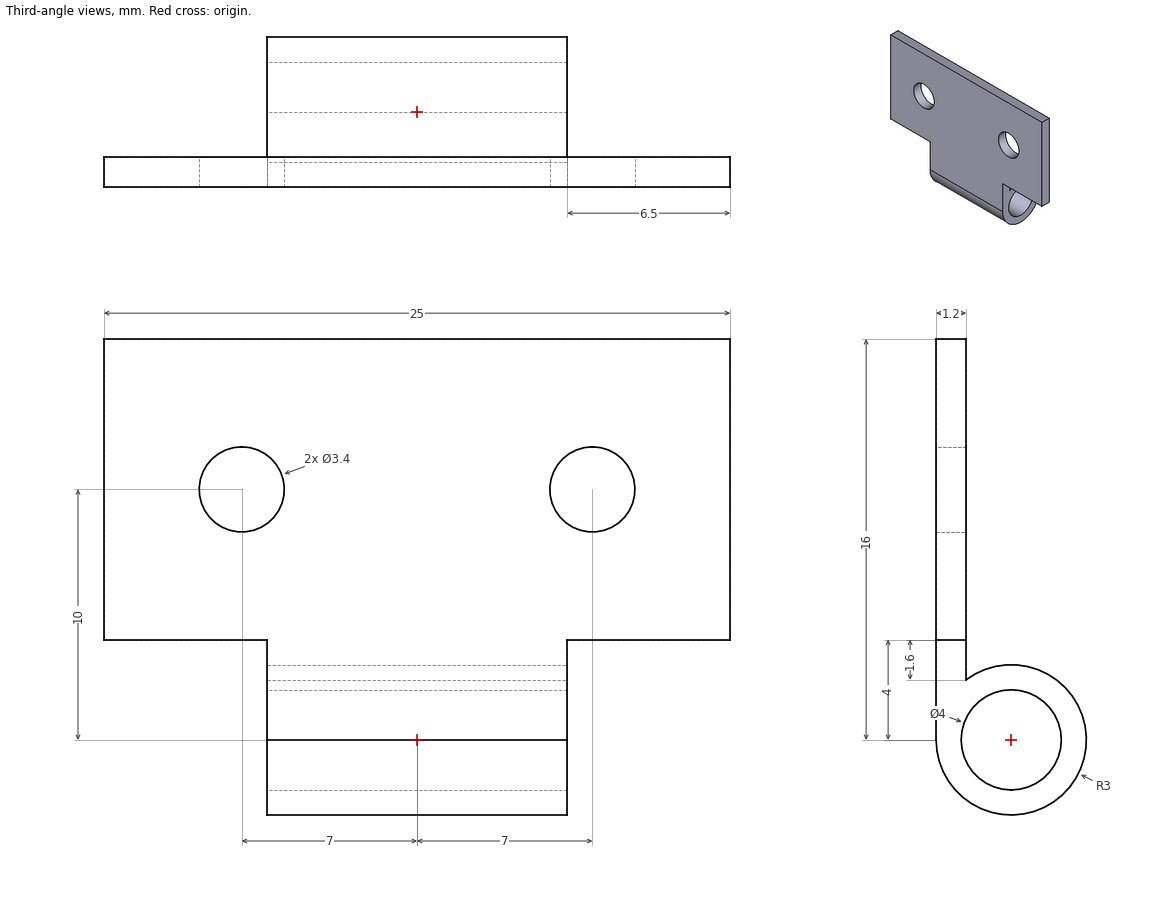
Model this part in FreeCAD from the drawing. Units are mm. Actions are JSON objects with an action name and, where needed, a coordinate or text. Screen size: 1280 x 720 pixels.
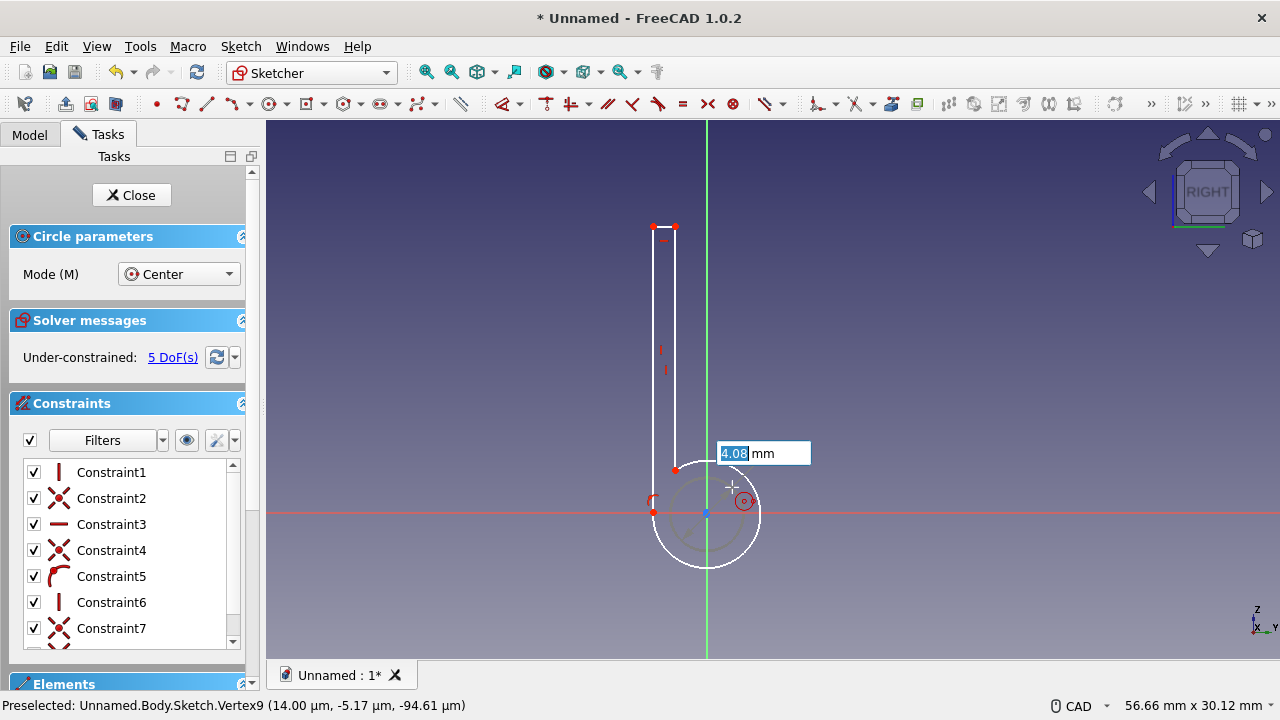
{"action": "type", "text": "4"}
{"action": "key", "text": "Return"}
{"action": "key", "text": "Escape"}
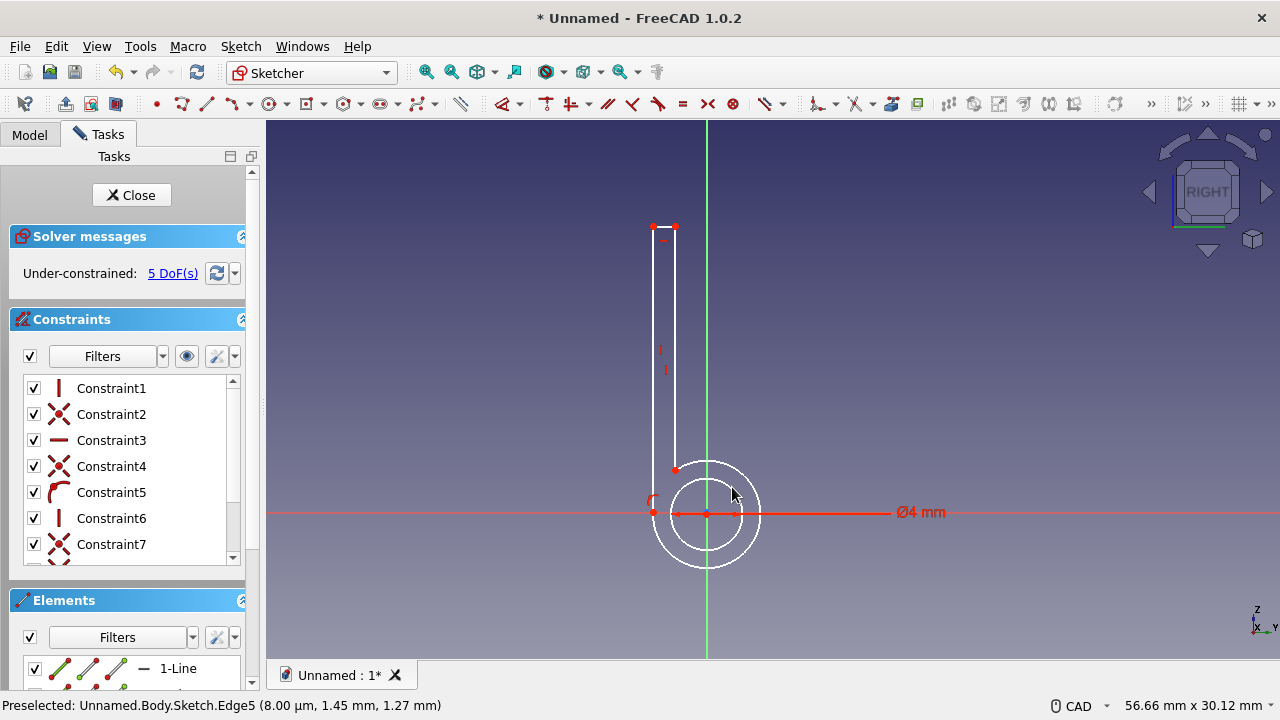
{"action": "left_click", "coordinate": [653, 313]}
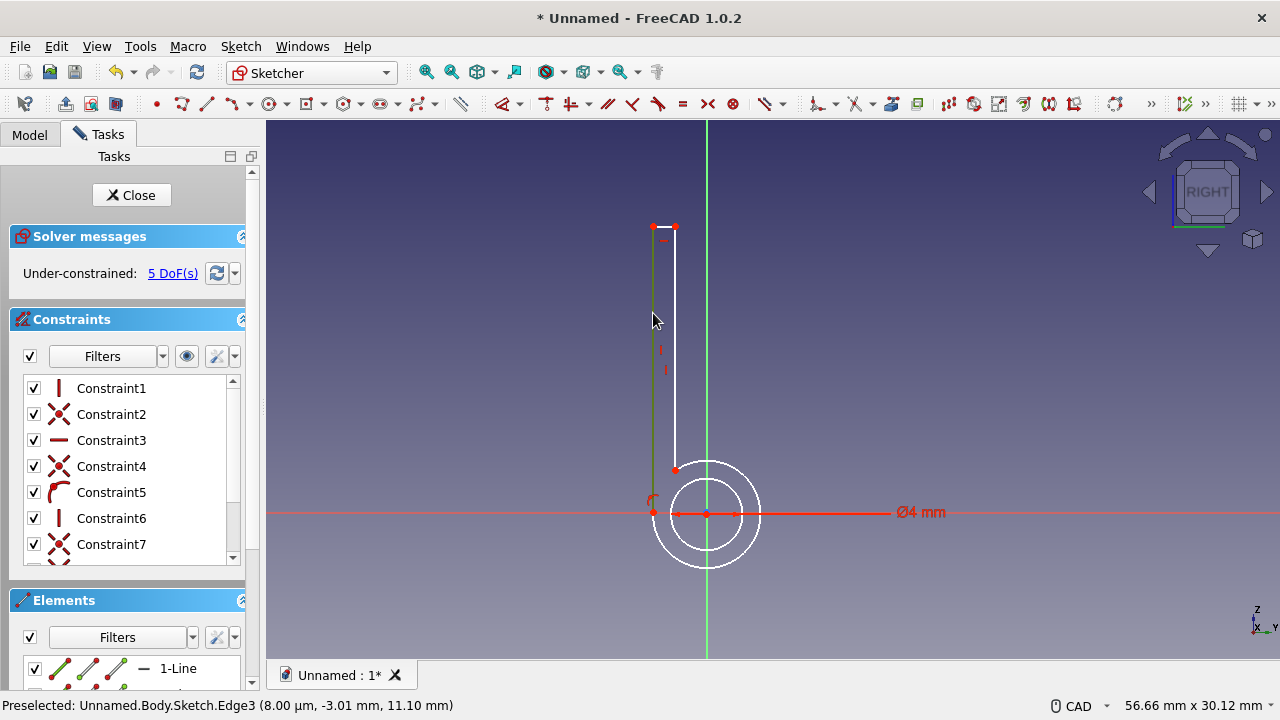
{"action": "left_click", "coordinate": [707, 568]}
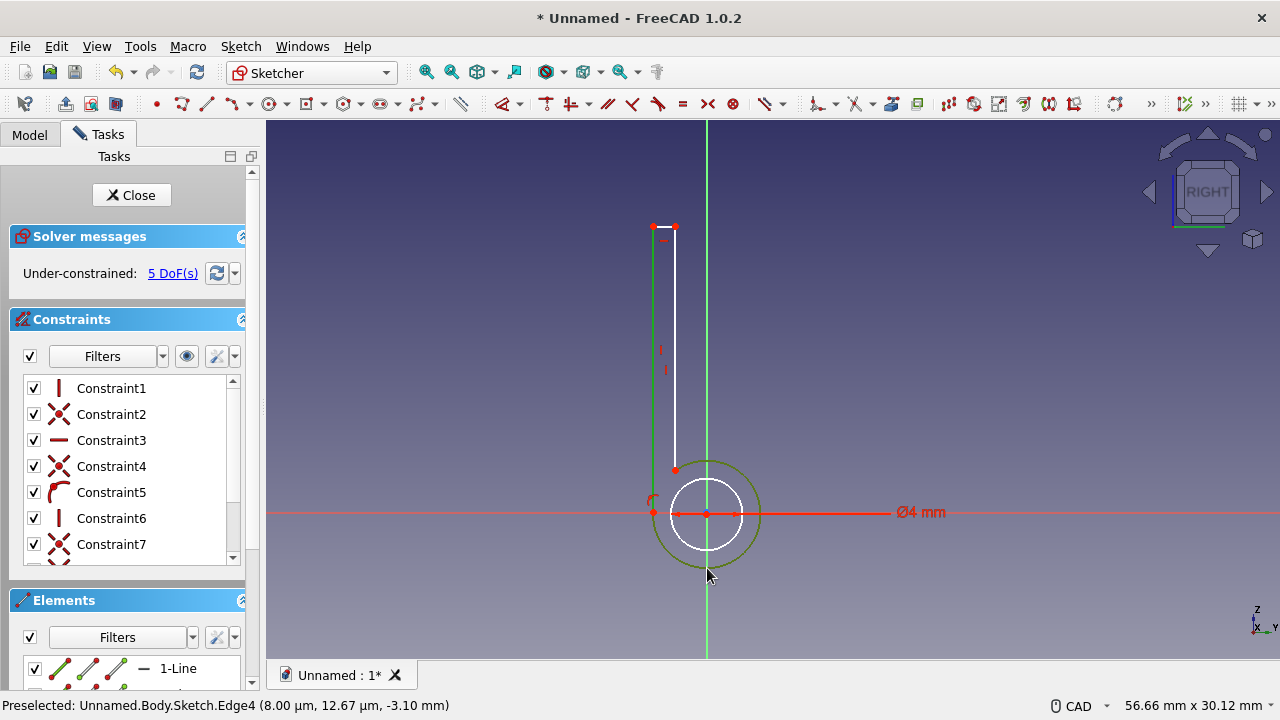
{"action": "left_click", "coordinate": [658, 104]}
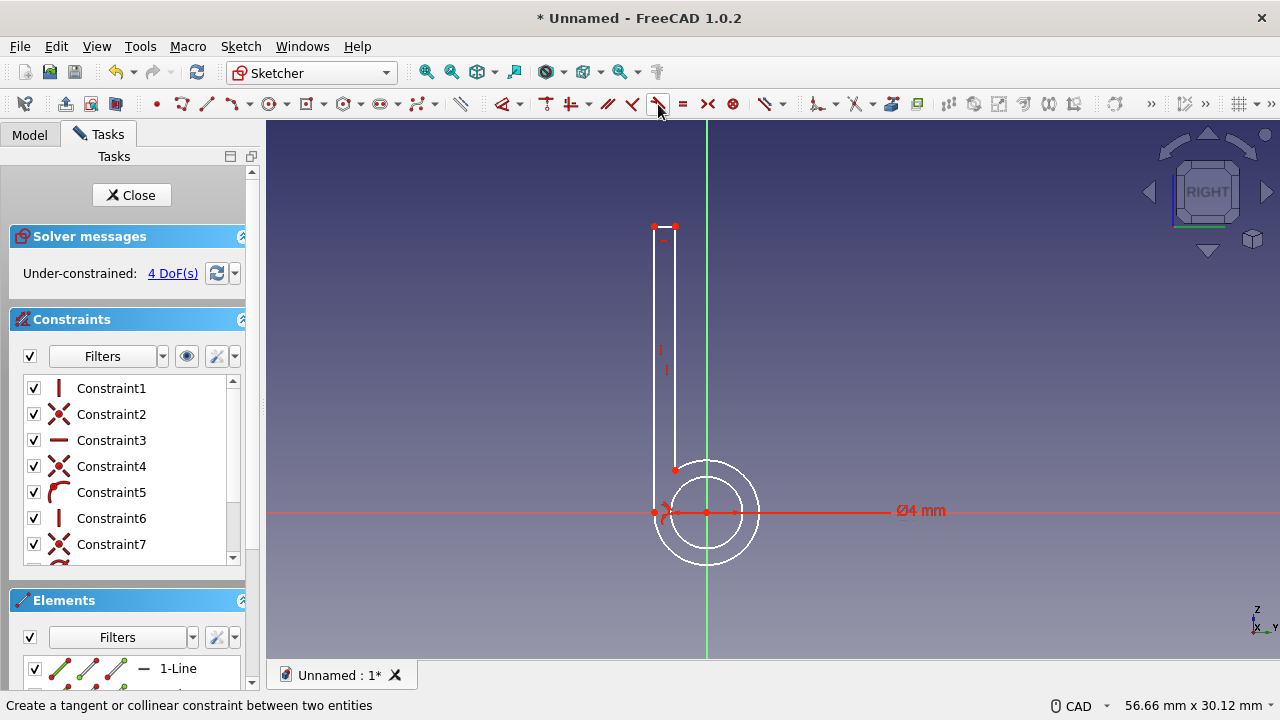
{"action": "left_click", "coordinate": [707, 513]}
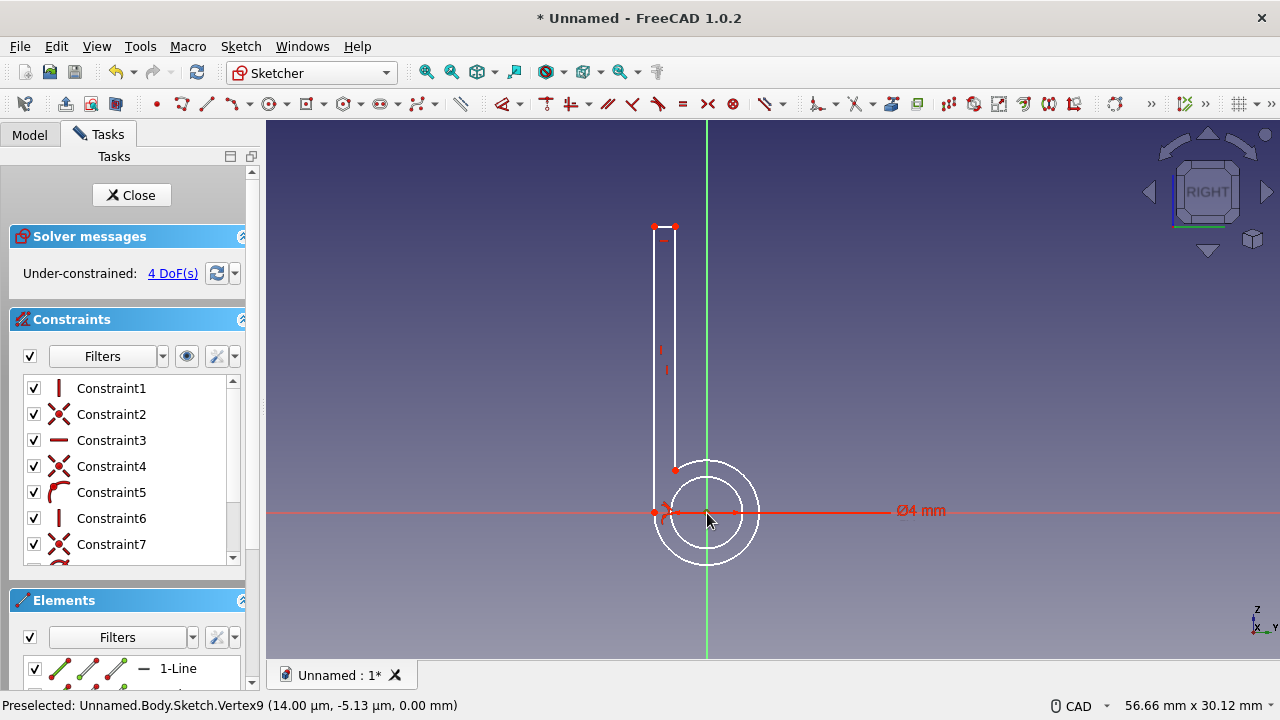
{"action": "left_click", "coordinate": [707, 596]}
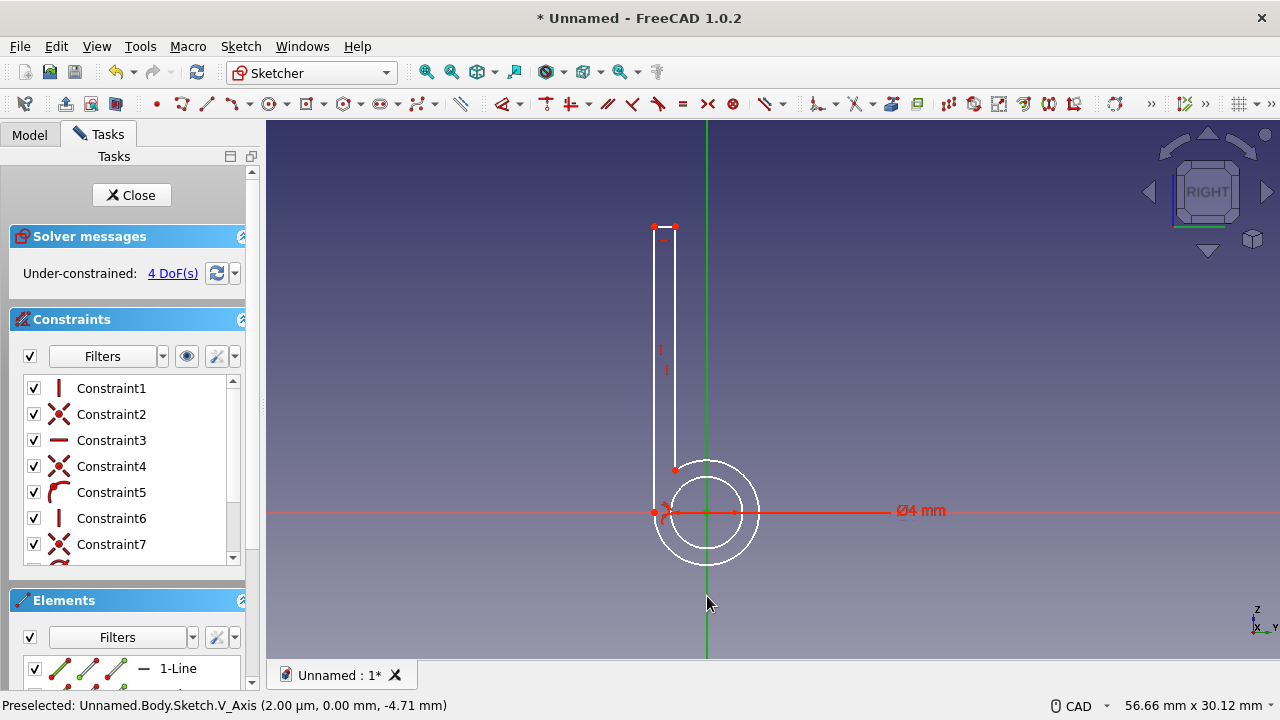
{"action": "left_click", "coordinate": [546, 104]}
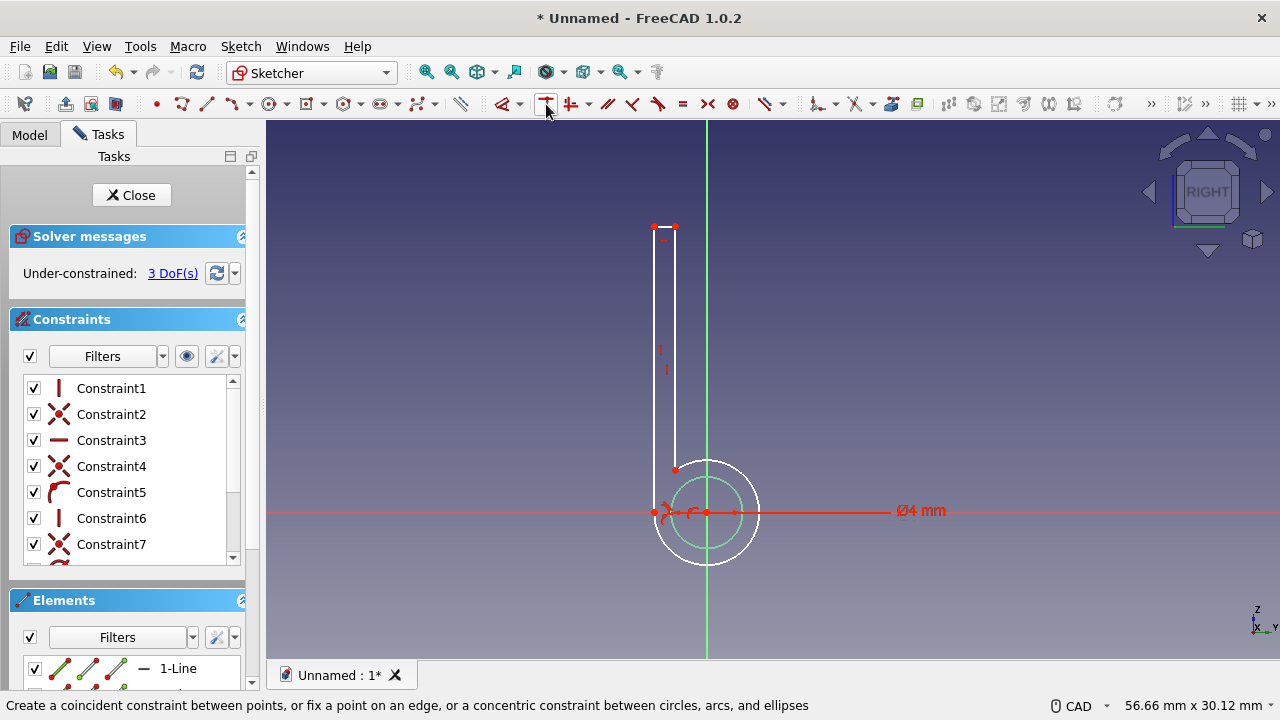
{"action": "left_click", "coordinate": [709, 565]}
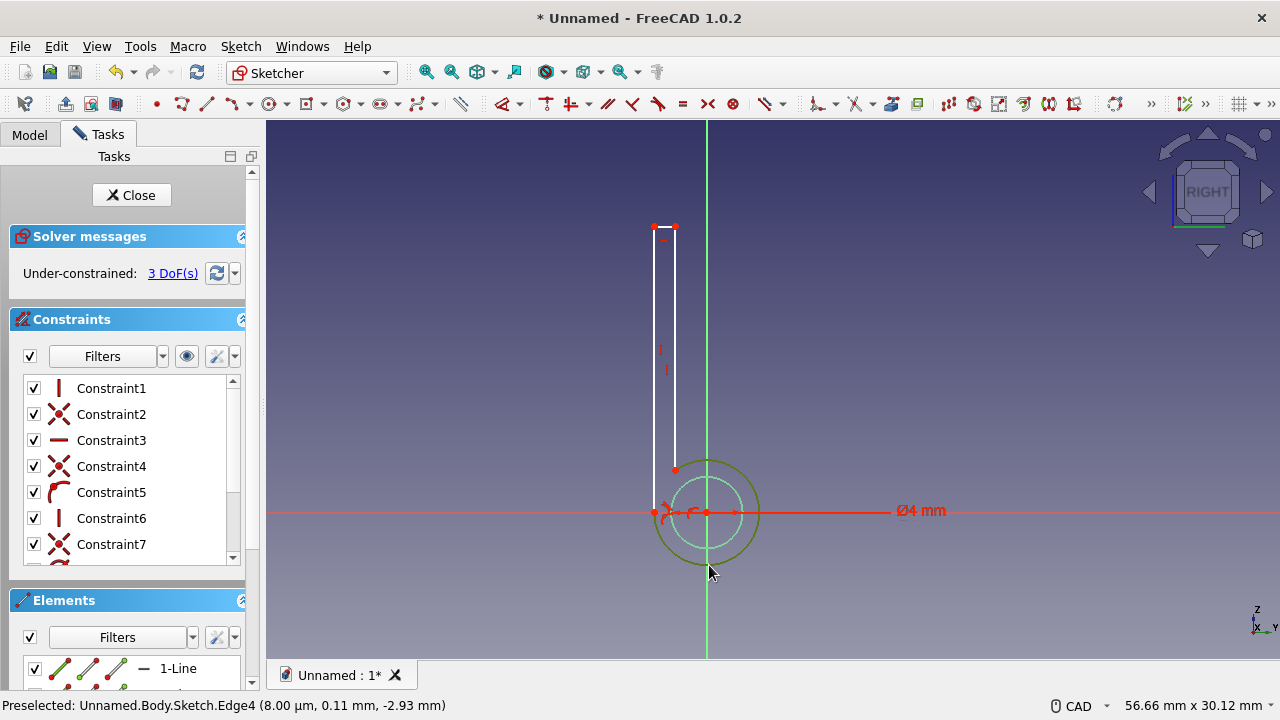
{"action": "left_click", "coordinate": [520, 104]}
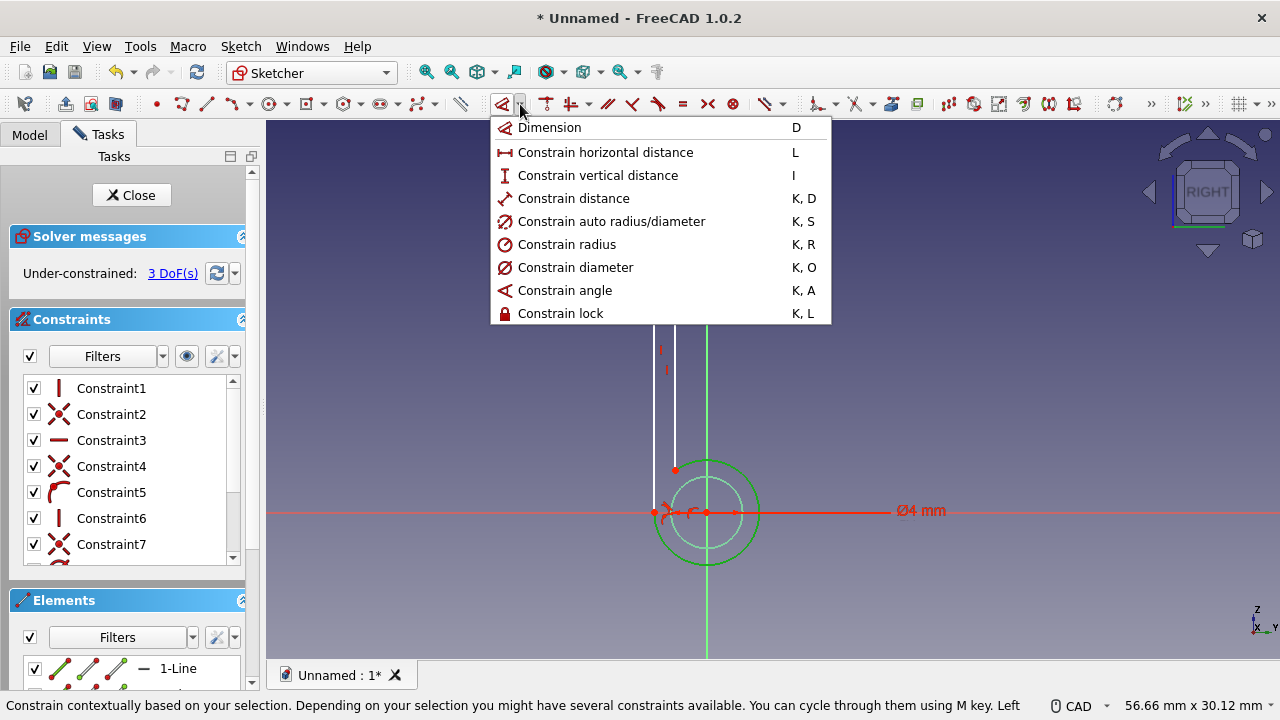
{"action": "left_click", "coordinate": [661, 244]}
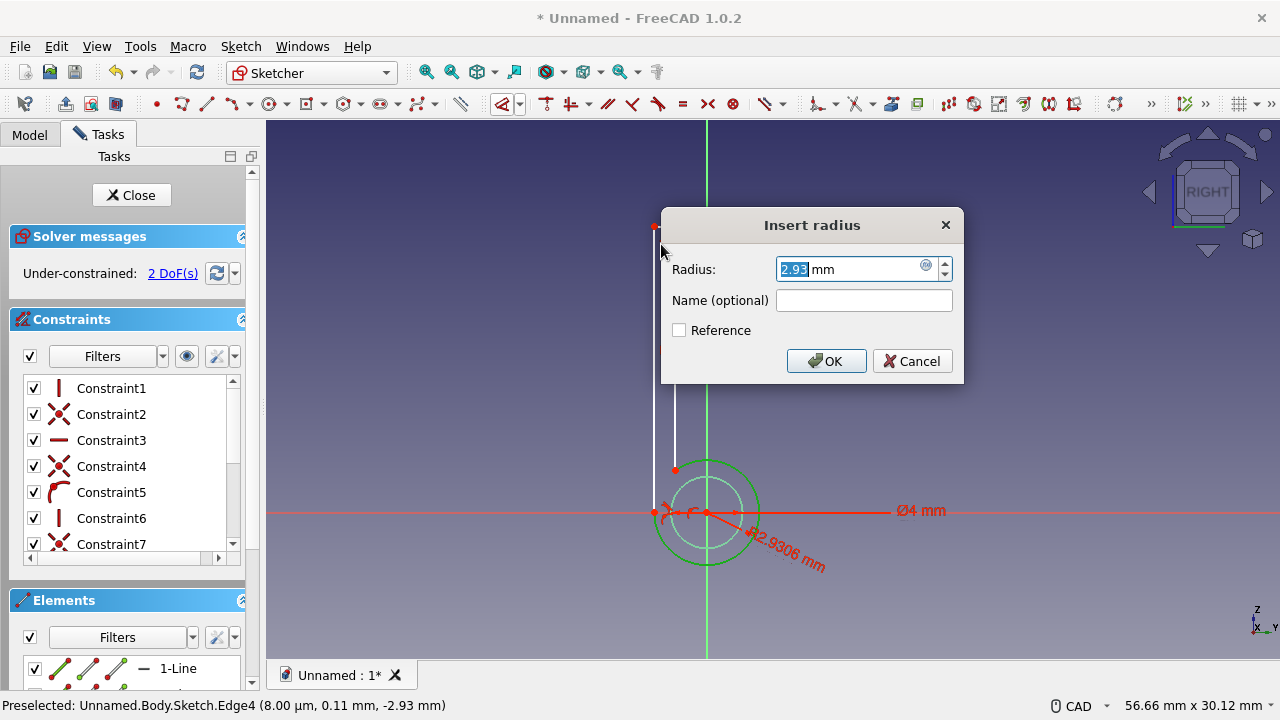
{"action": "type", "text": "3"}
{"action": "key", "text": "Return"}